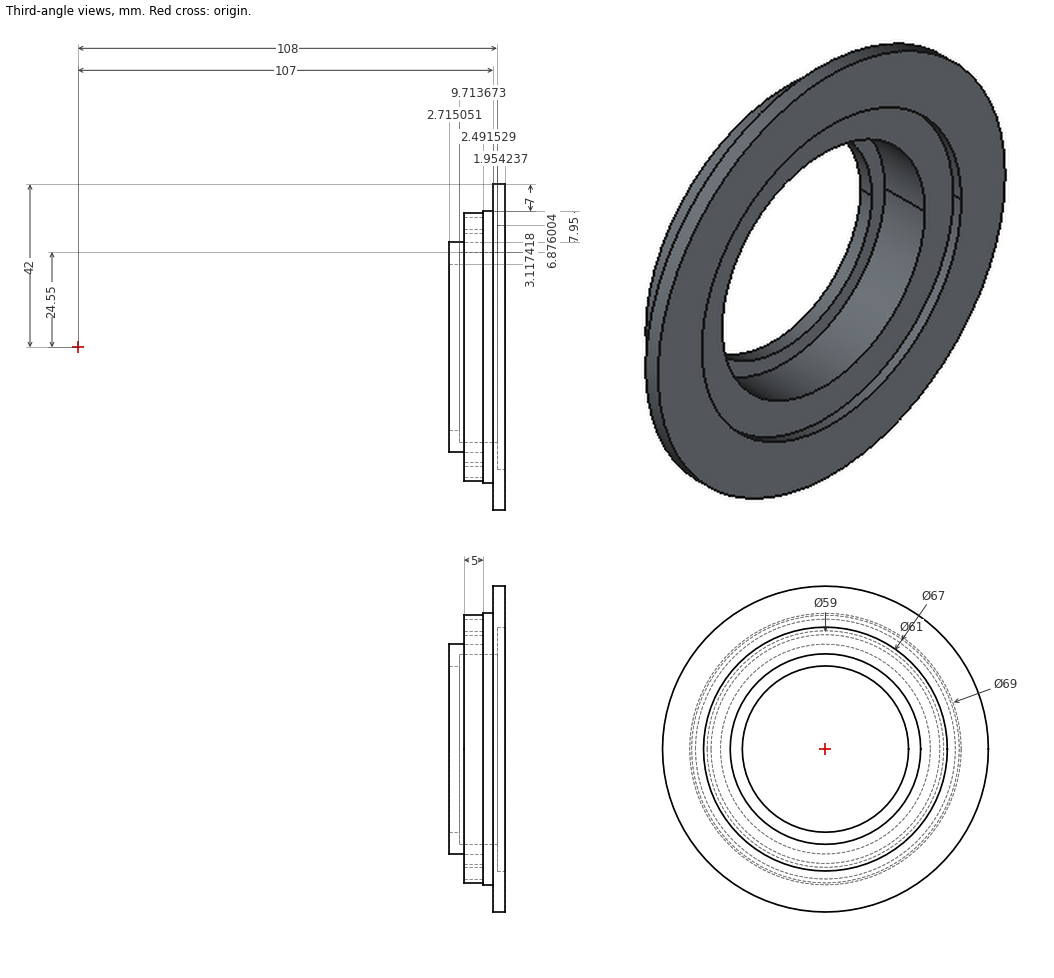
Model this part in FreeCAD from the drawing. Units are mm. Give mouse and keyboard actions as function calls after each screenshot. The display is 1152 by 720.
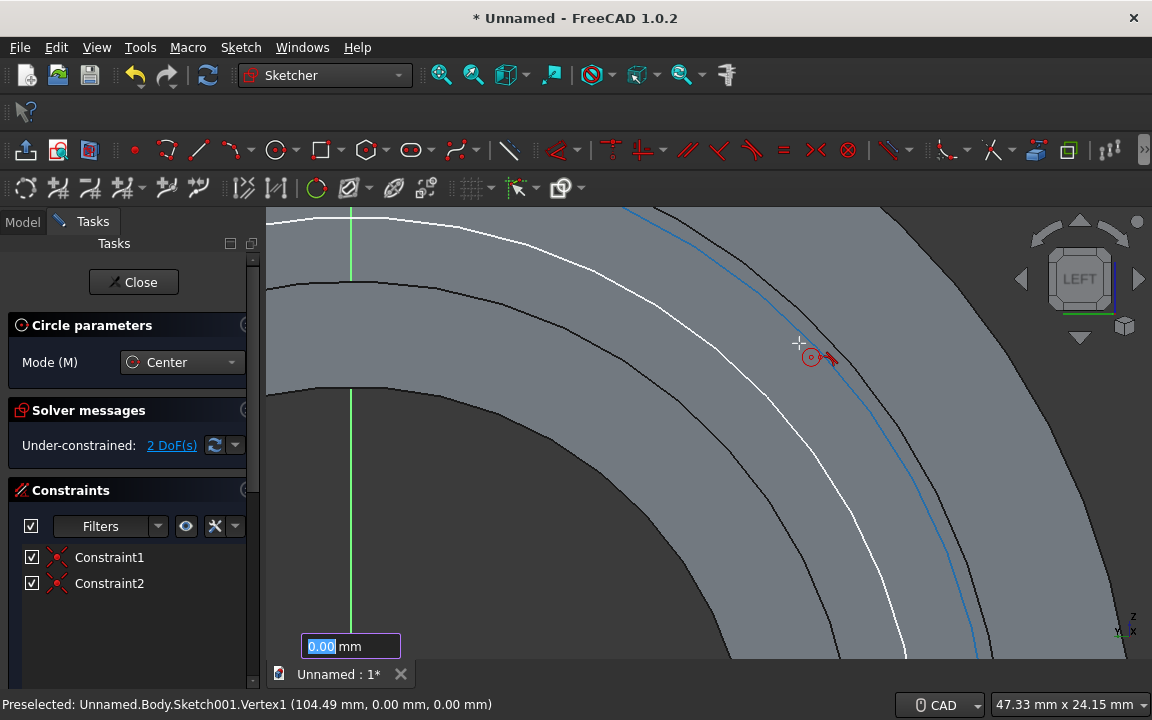
click(795, 344)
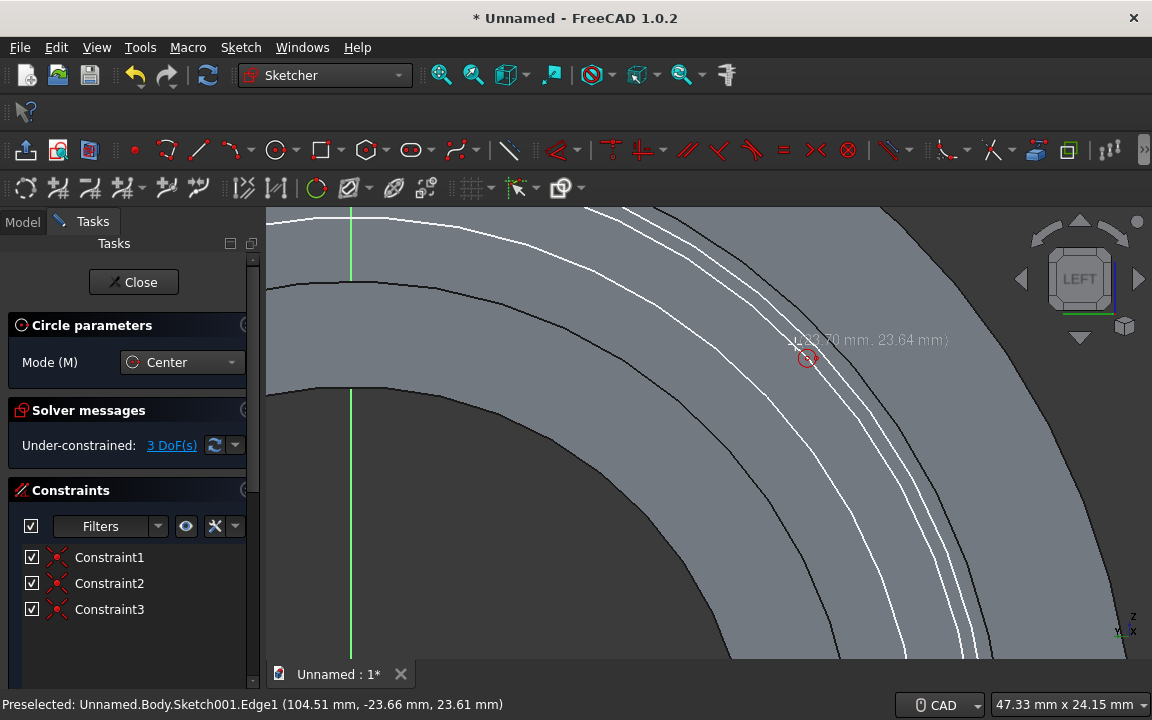
scroll(714, 343, down, 8)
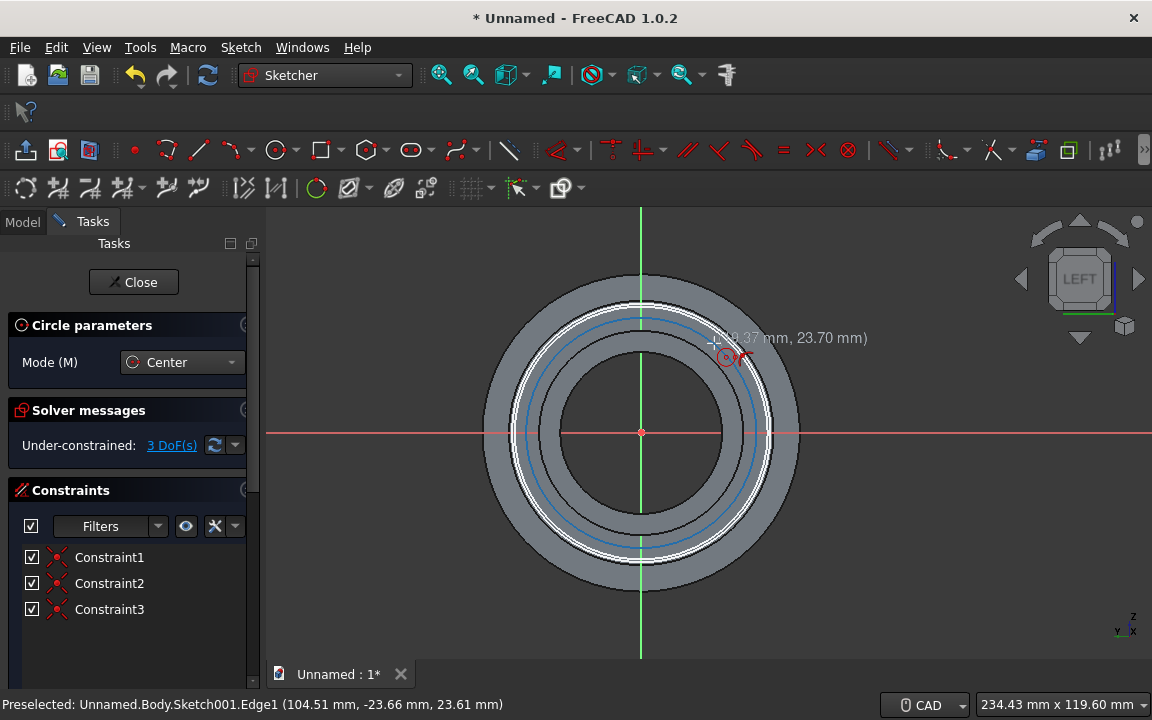
click(641, 433)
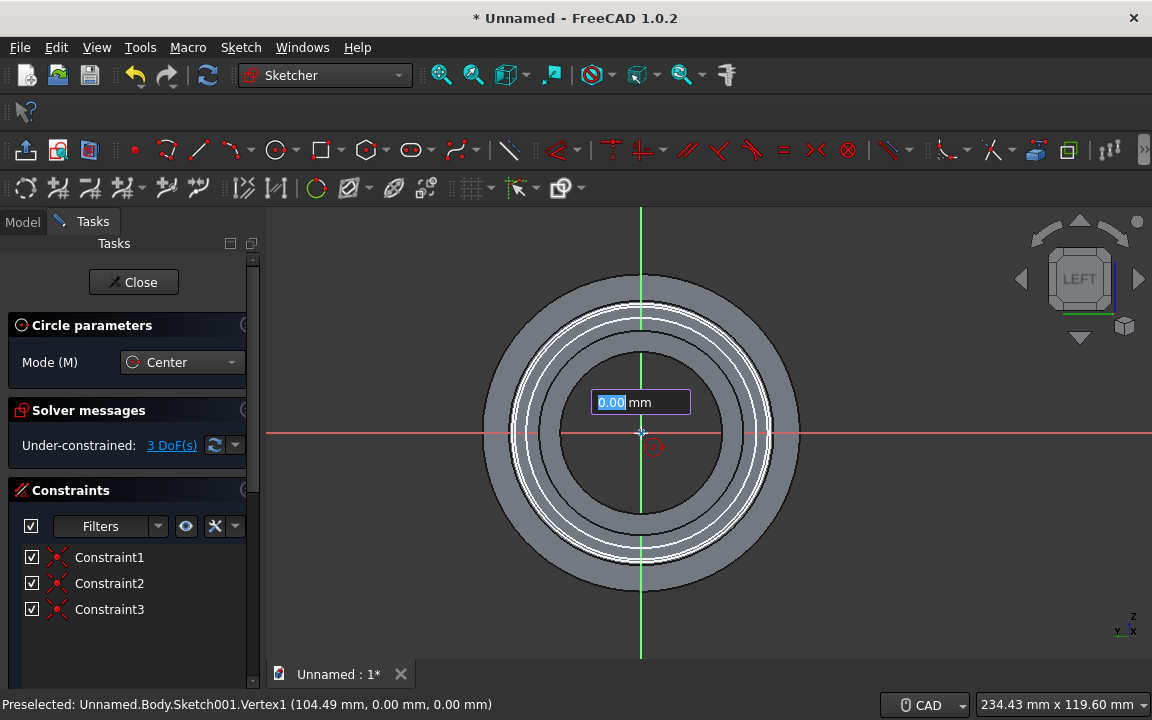
scroll(720, 354, up, 8)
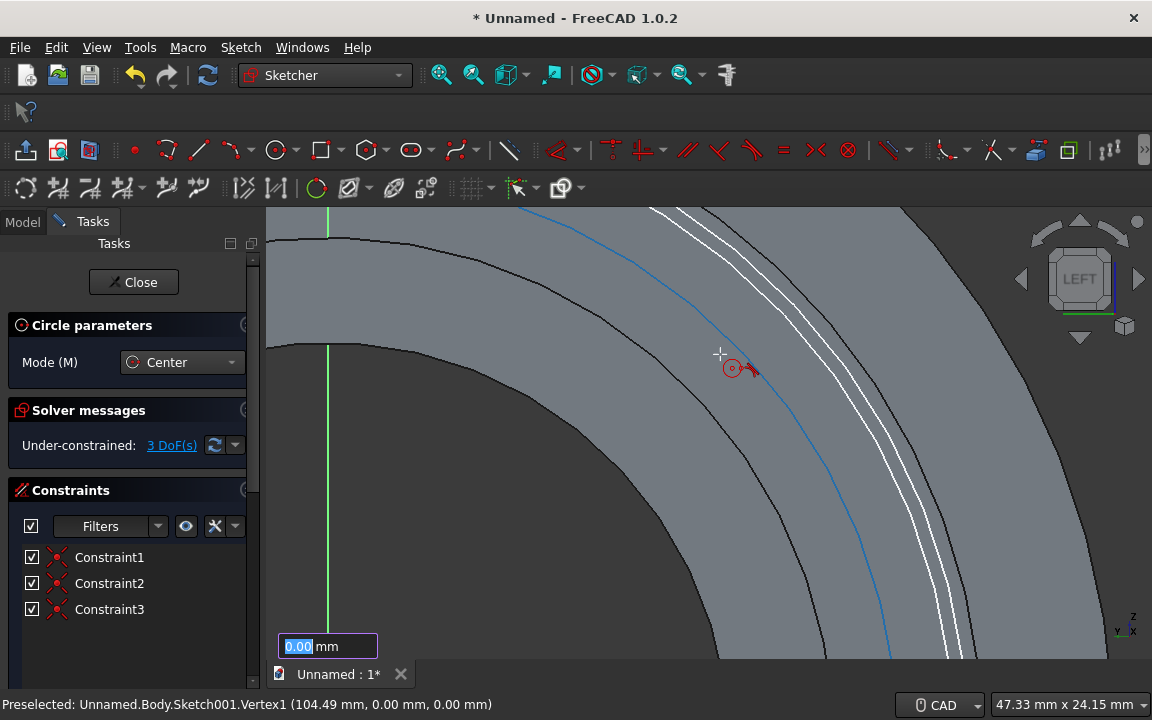
click(718, 354)
key(Escape)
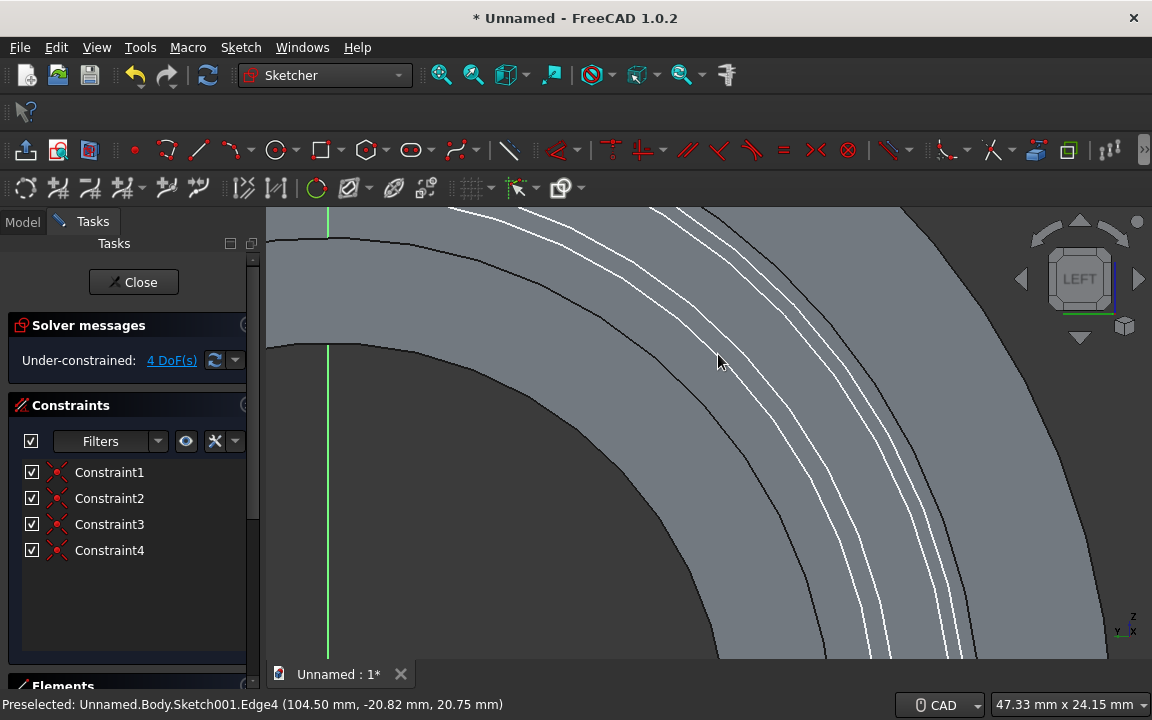
click(556, 150)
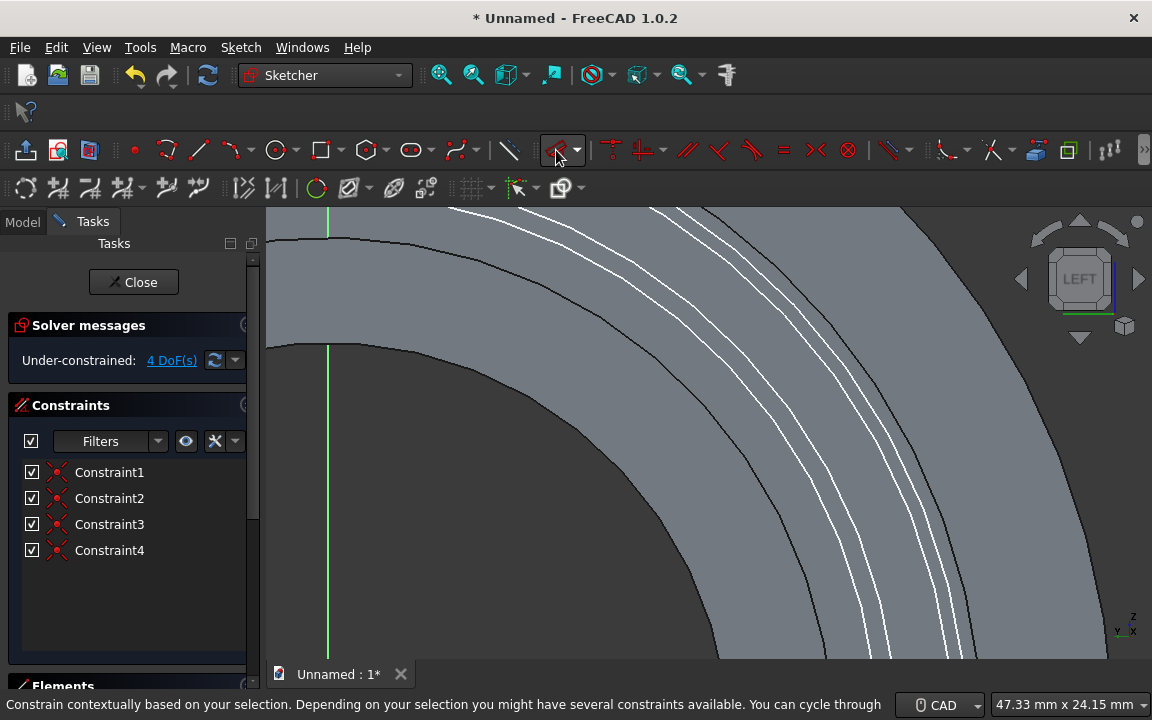
click(779, 290)
click(802, 267)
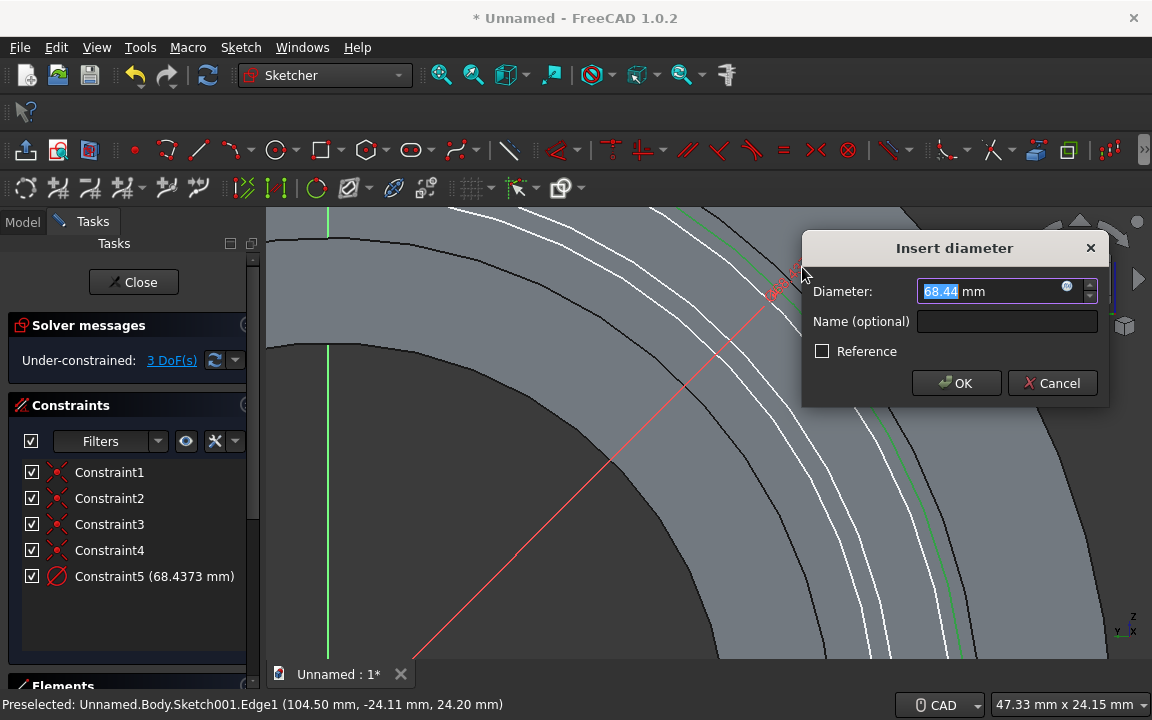
text(69)
key(Return)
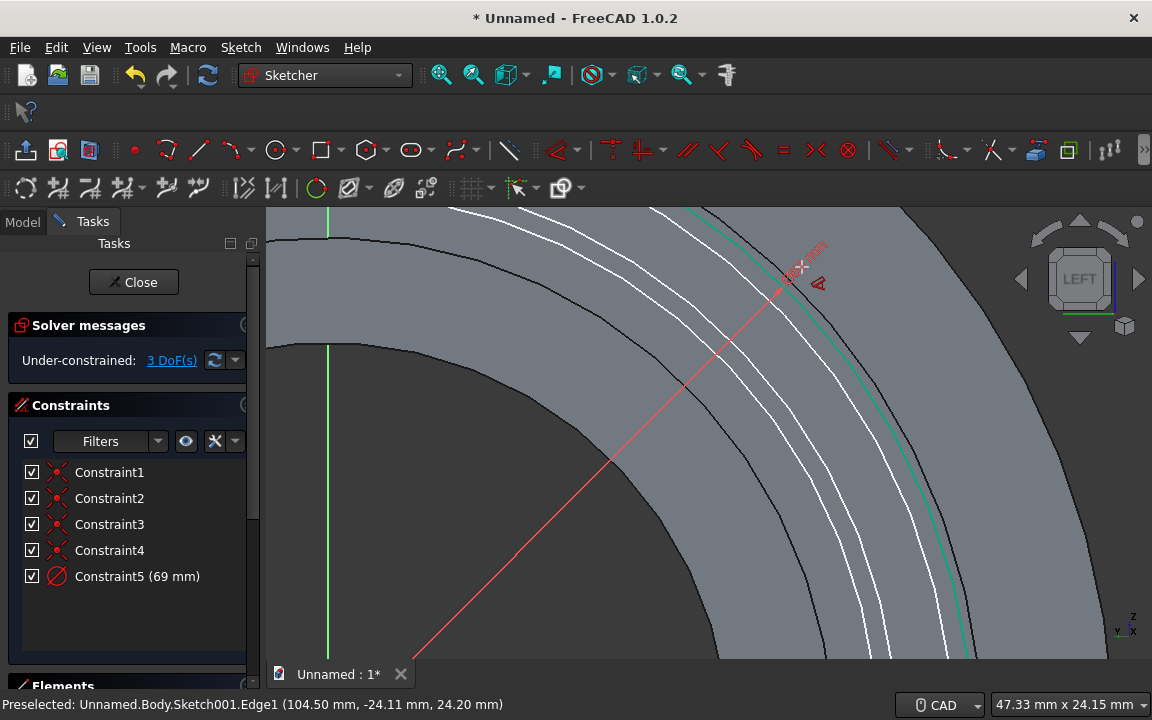
click(730, 339)
click(753, 316)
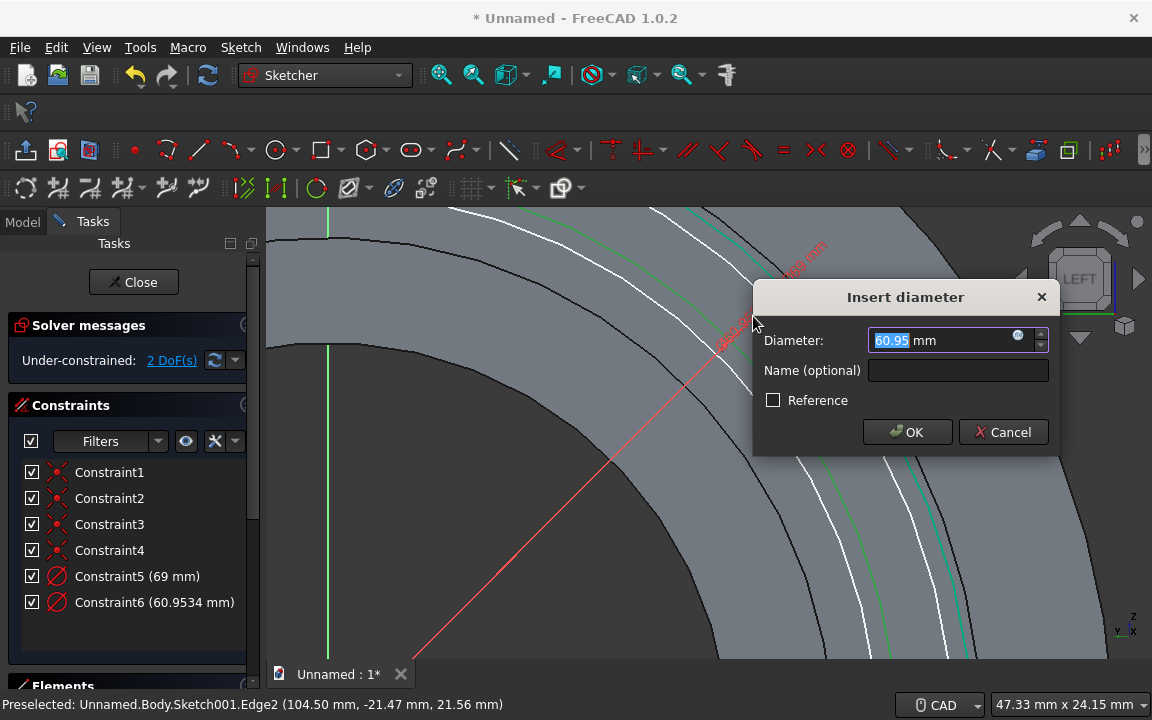
text(61)
key(Return)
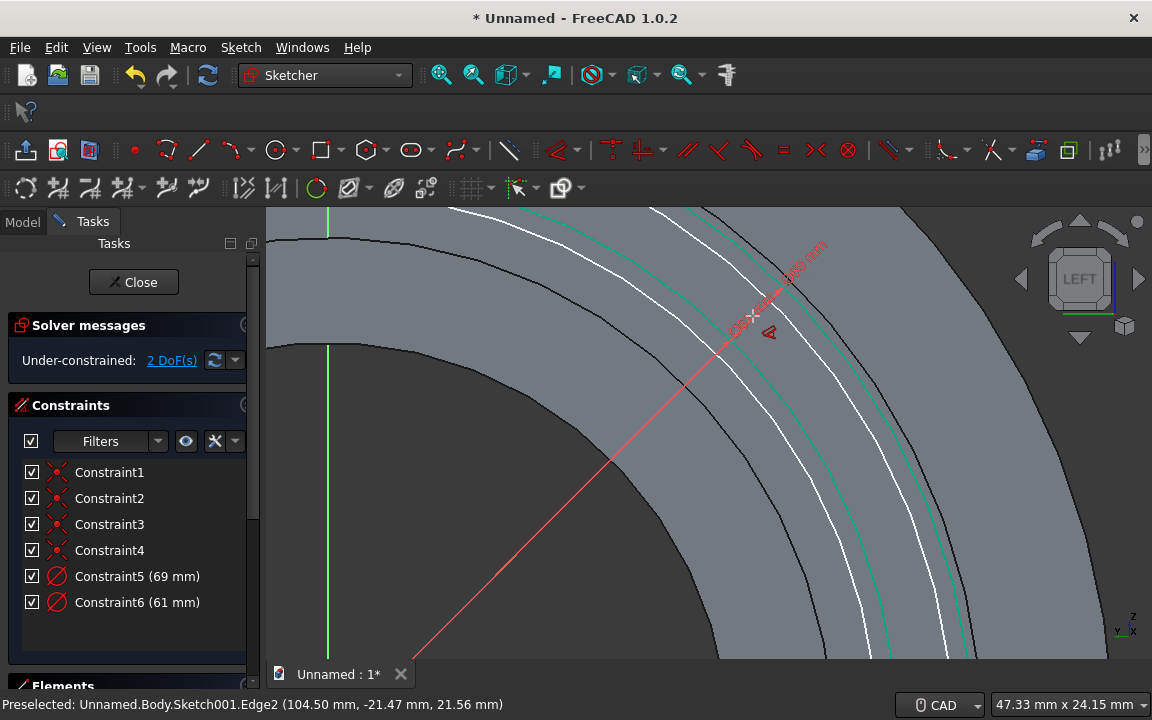
click(769, 300)
click(981, 550)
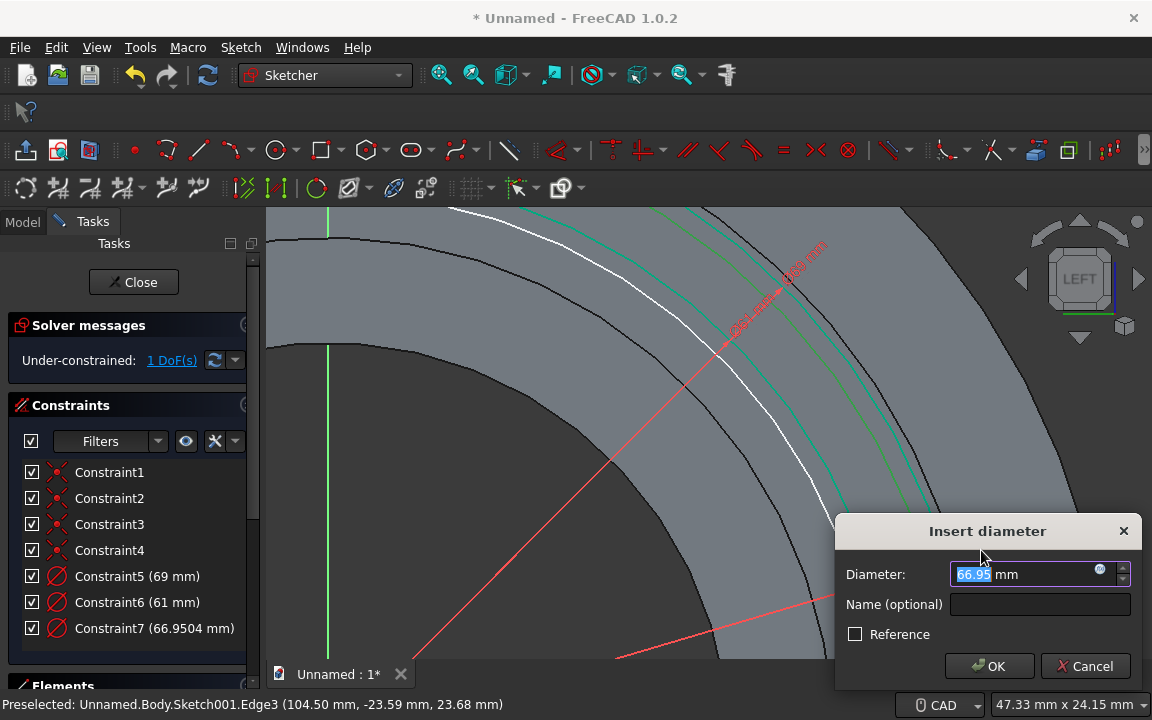
text(67)
key(Return)